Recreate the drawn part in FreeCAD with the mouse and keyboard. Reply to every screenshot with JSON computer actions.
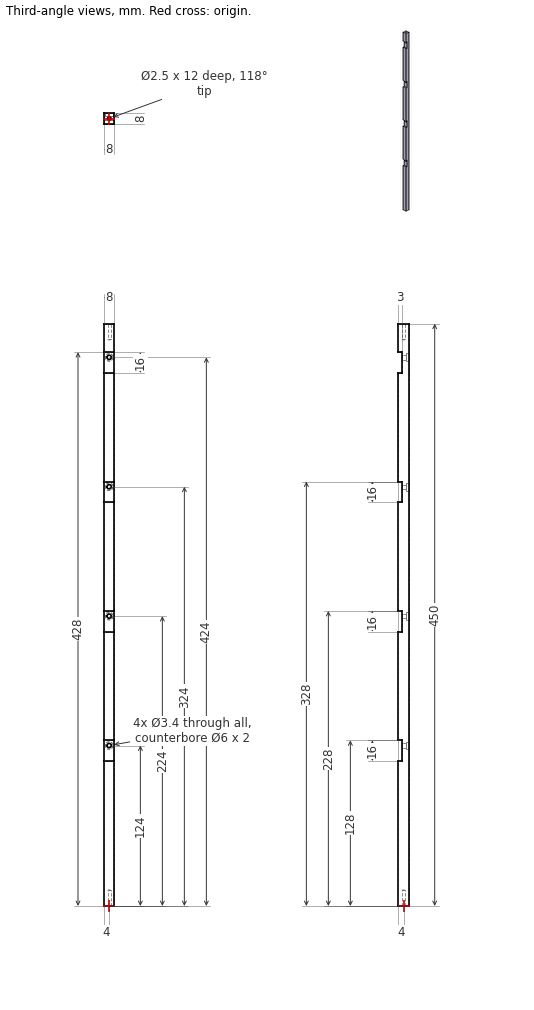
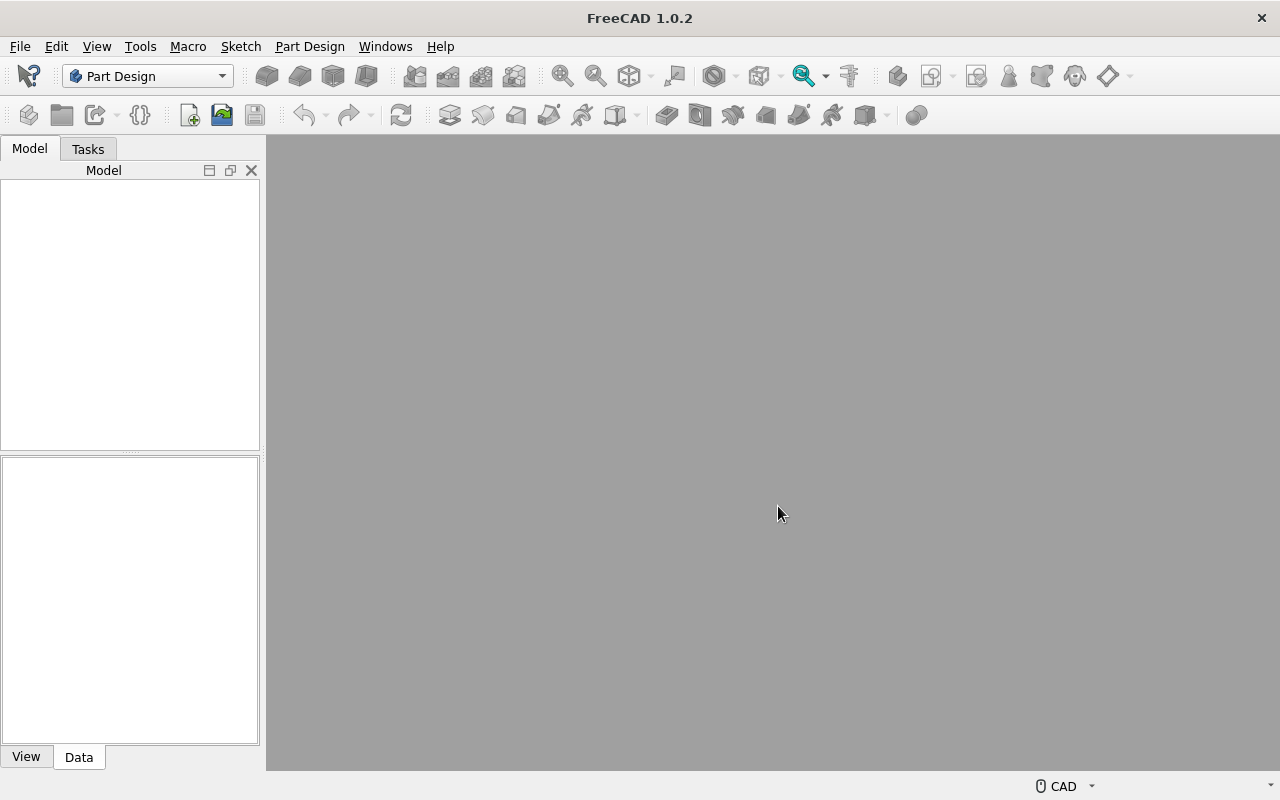
{"action": "key", "text": "ctrl+n"}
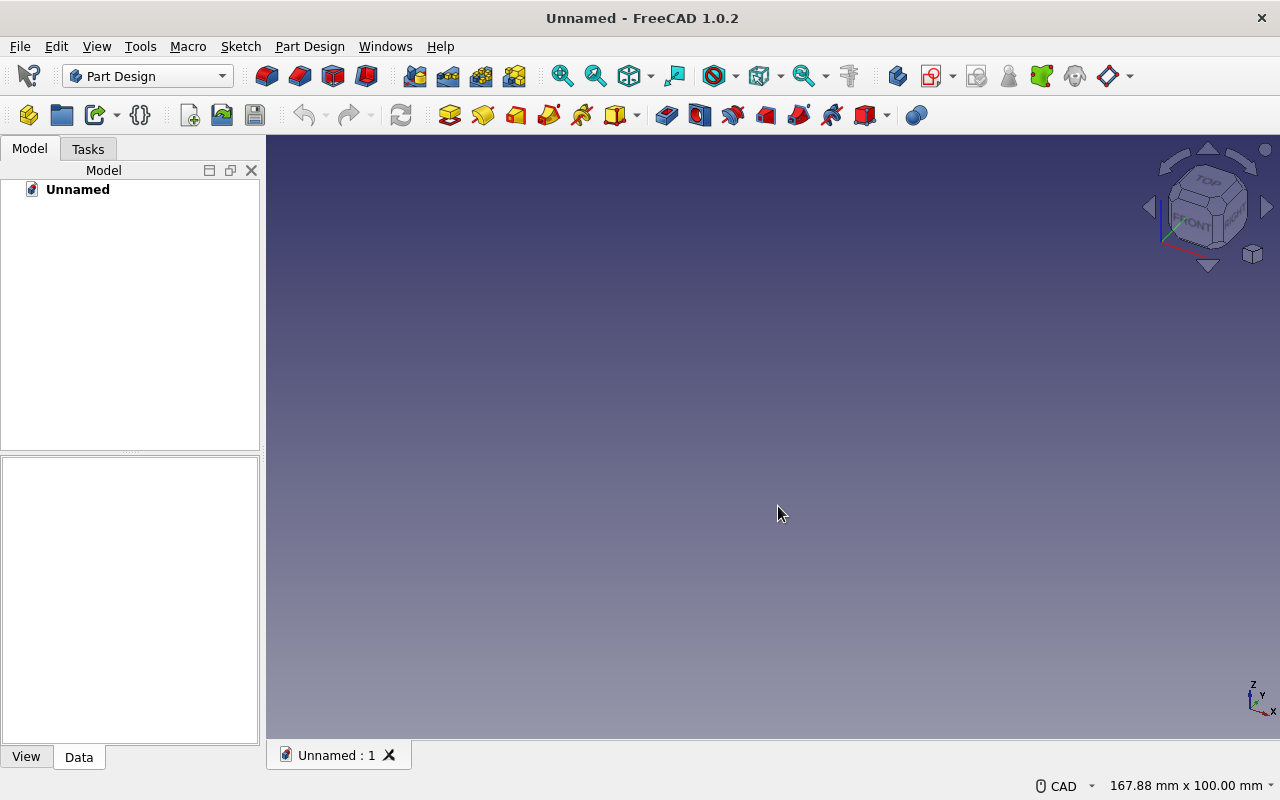
{"action": "left_click", "coordinate": [930, 76]}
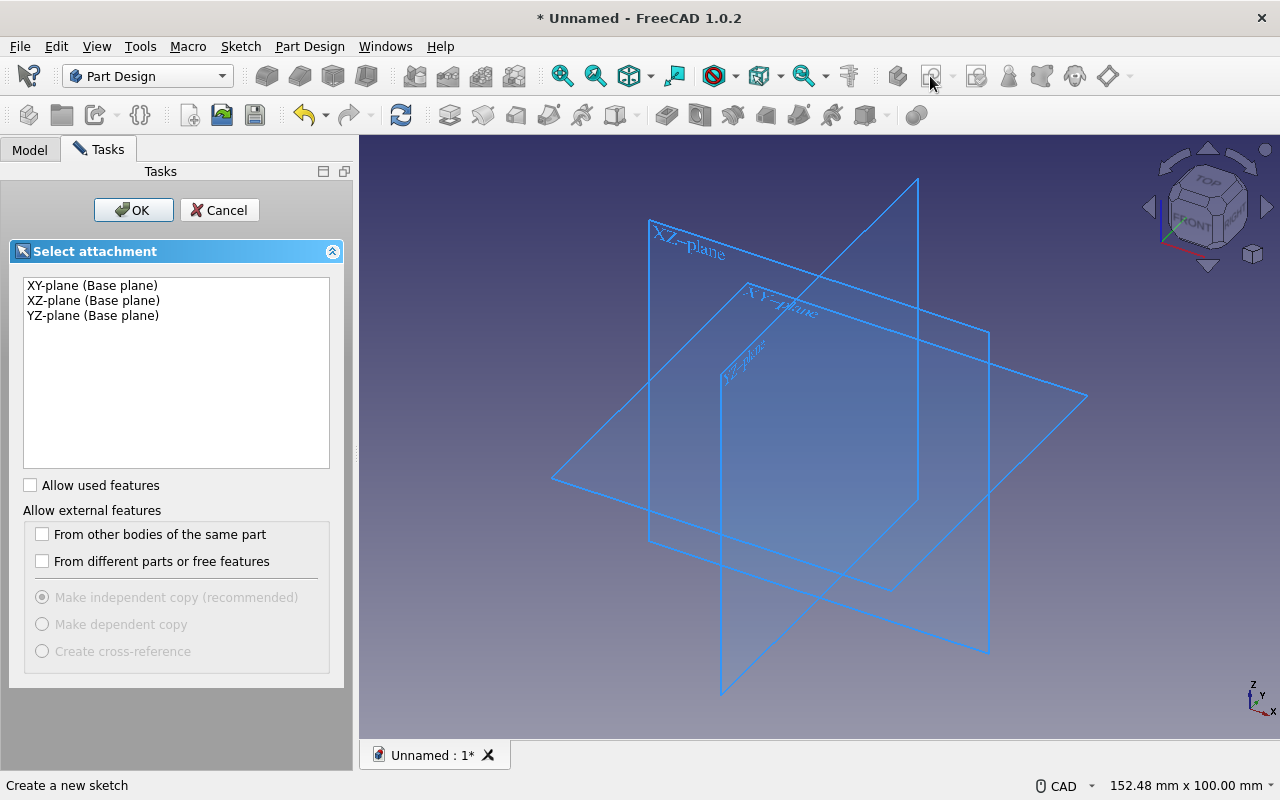
{"action": "left_click", "coordinate": [84, 286]}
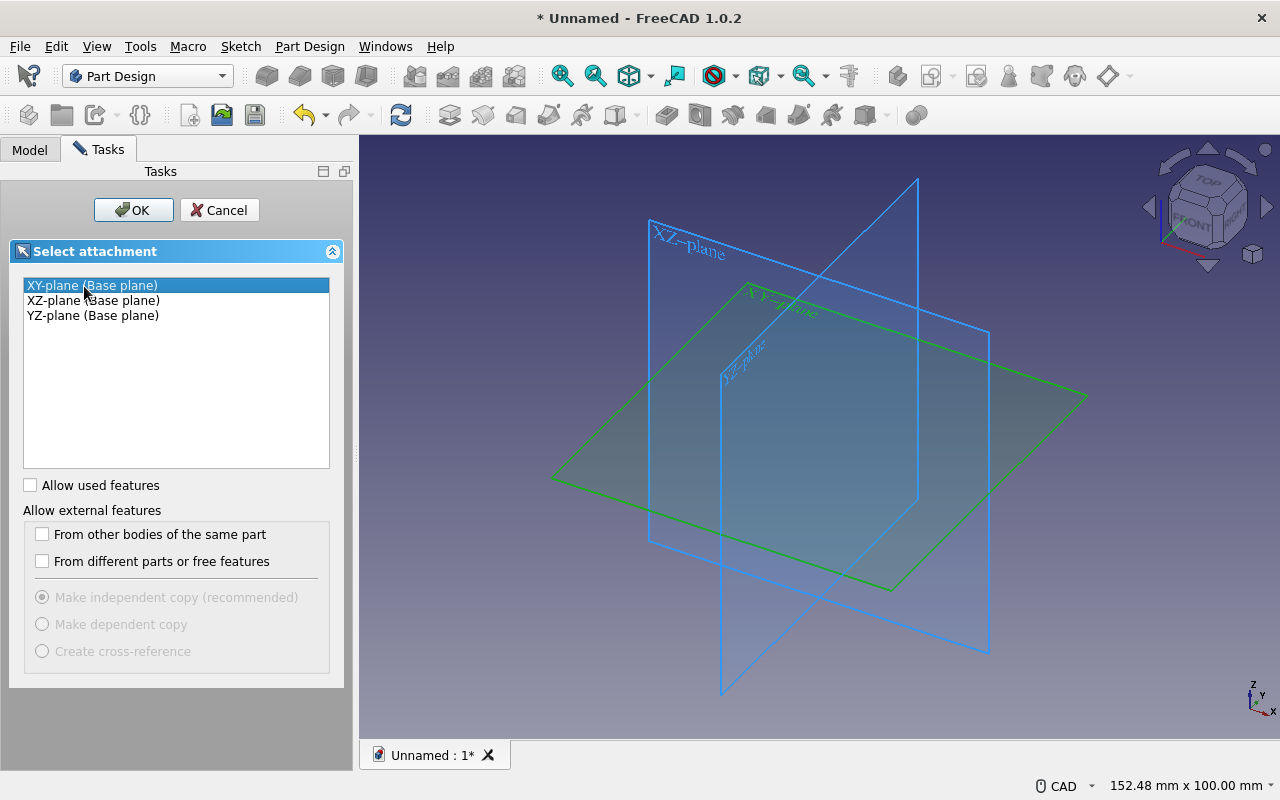
{"action": "left_click", "coordinate": [134, 210]}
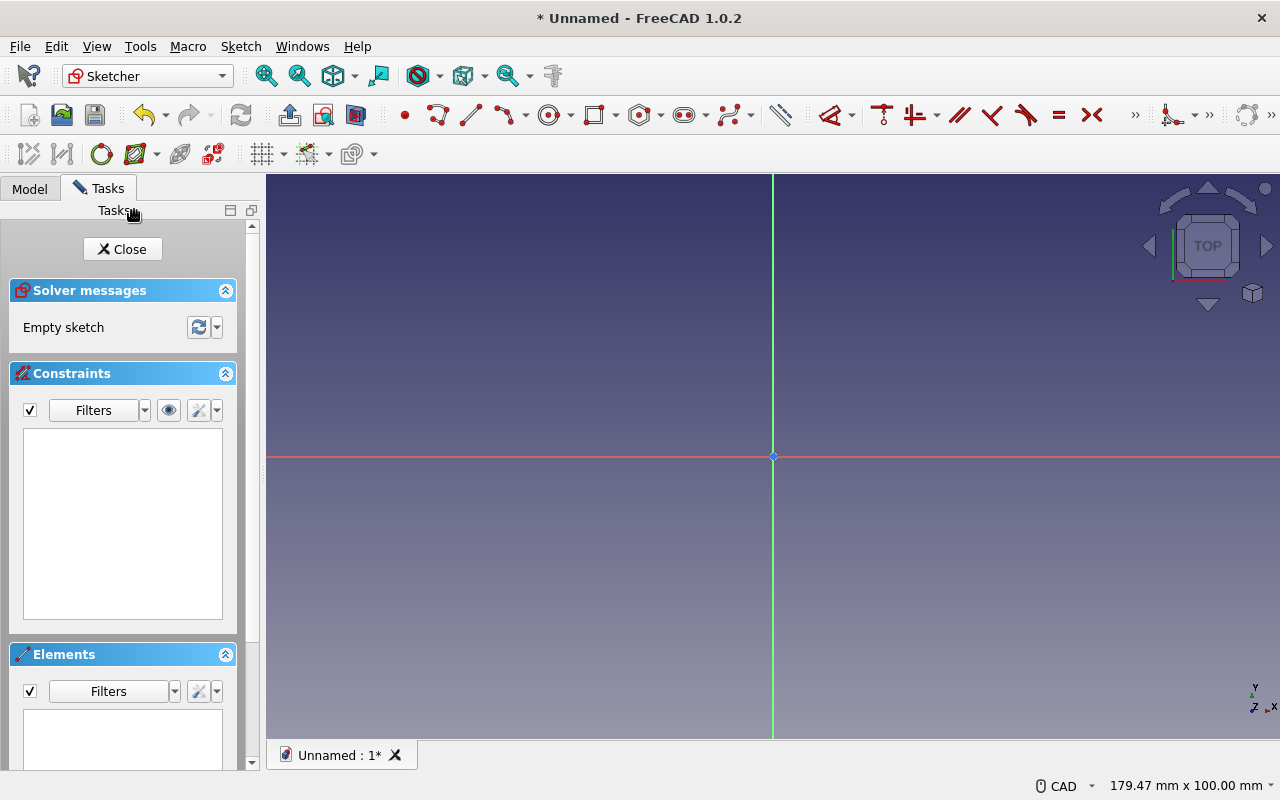
{"action": "scroll", "coordinate": [784, 456], "scroll_direction": "up", "scroll_amount": 10}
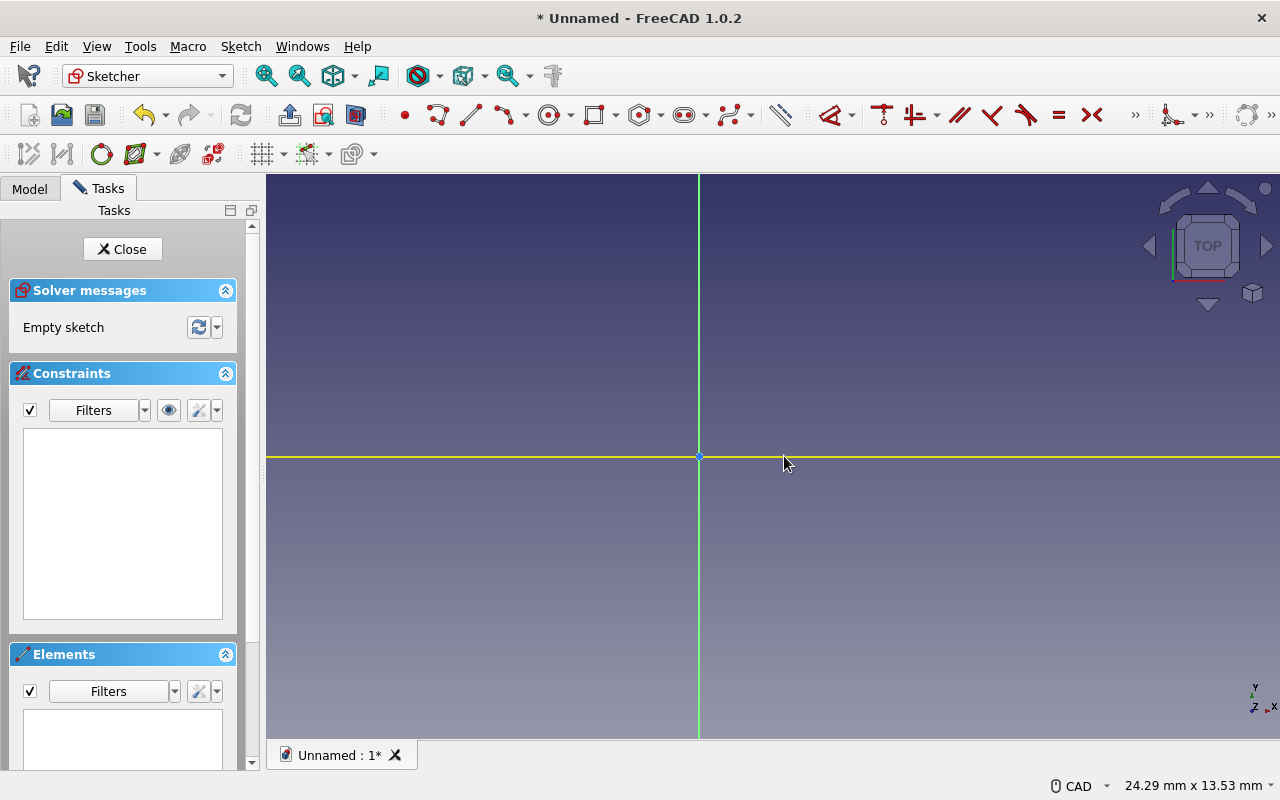
{"action": "key", "text": "g v"}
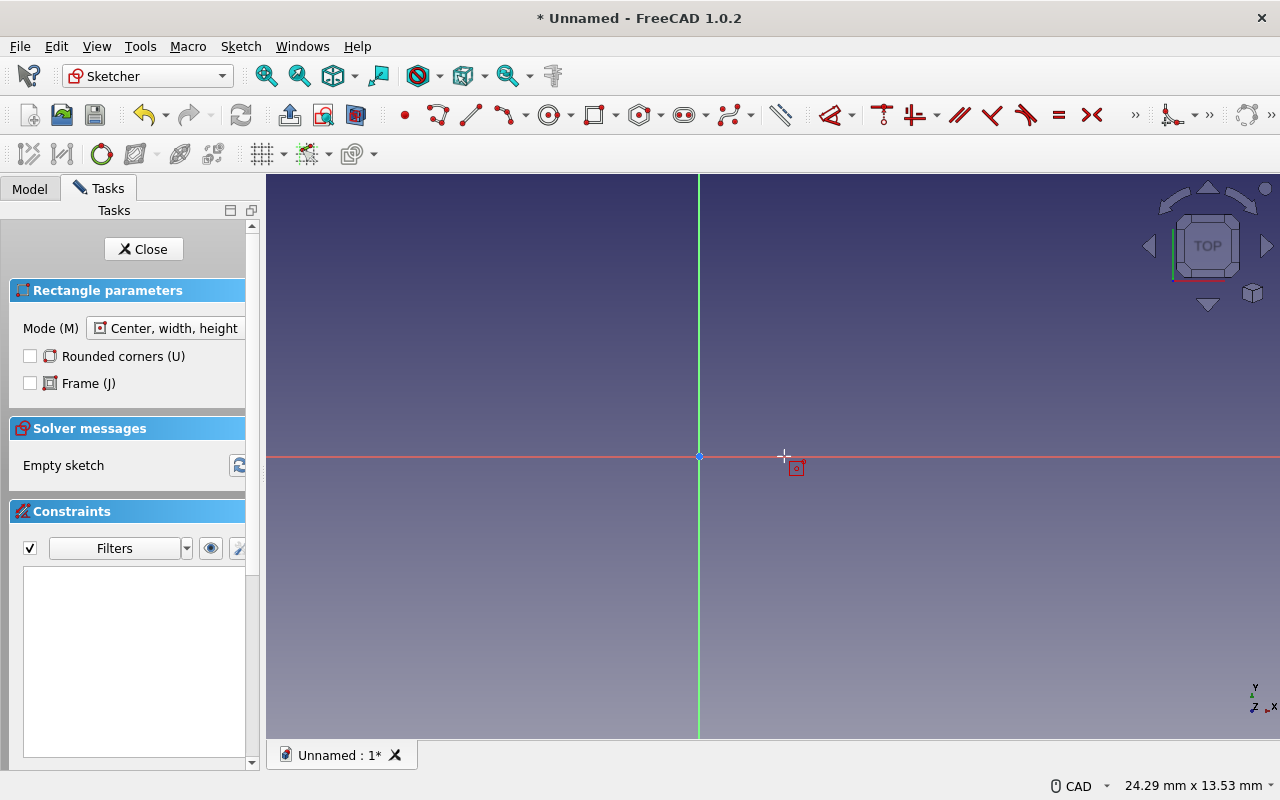
{"action": "left_click", "coordinate": [699, 456]}
{"action": "mouse_move", "coordinate": [866, 290]}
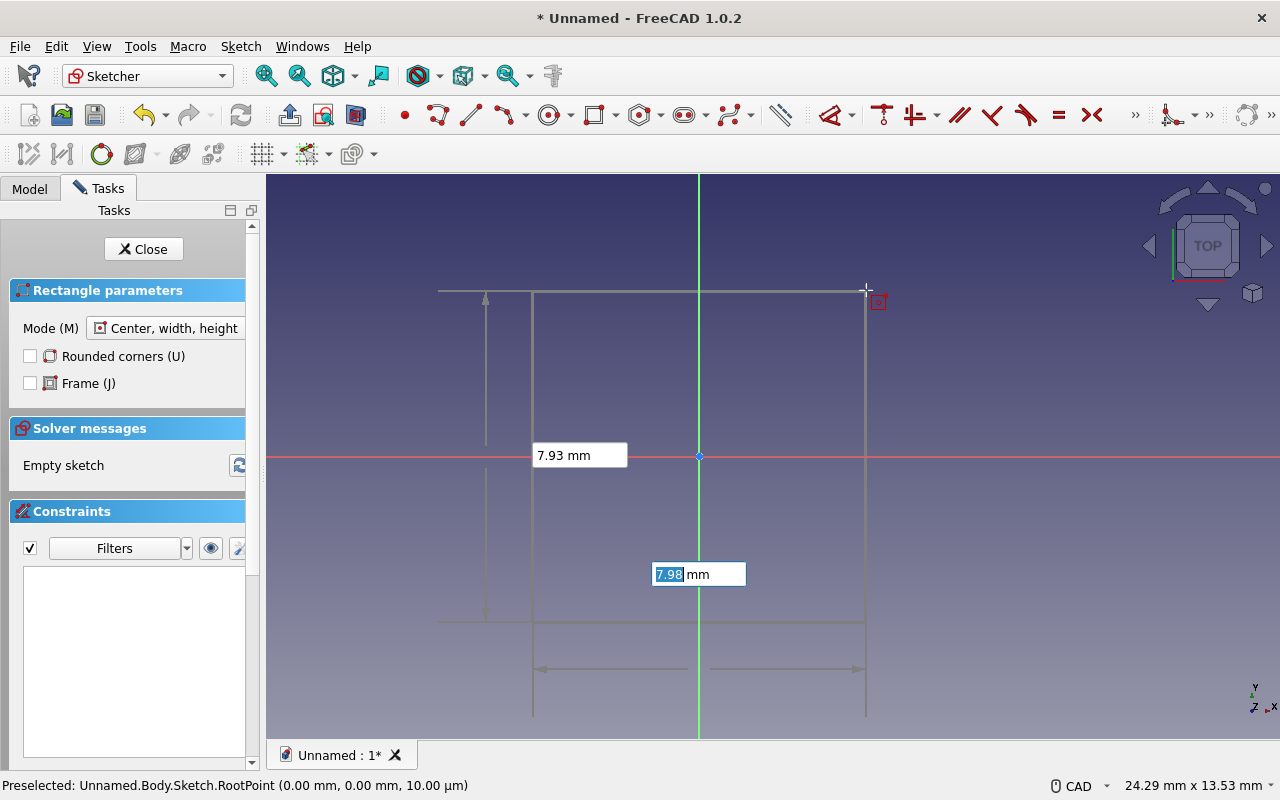
{"action": "type", "text": "8"}
{"action": "key", "text": "Tab"}
{"action": "type", "text": "8"}
{"action": "key", "text": "Return"}
{"action": "key", "text": "Escape"}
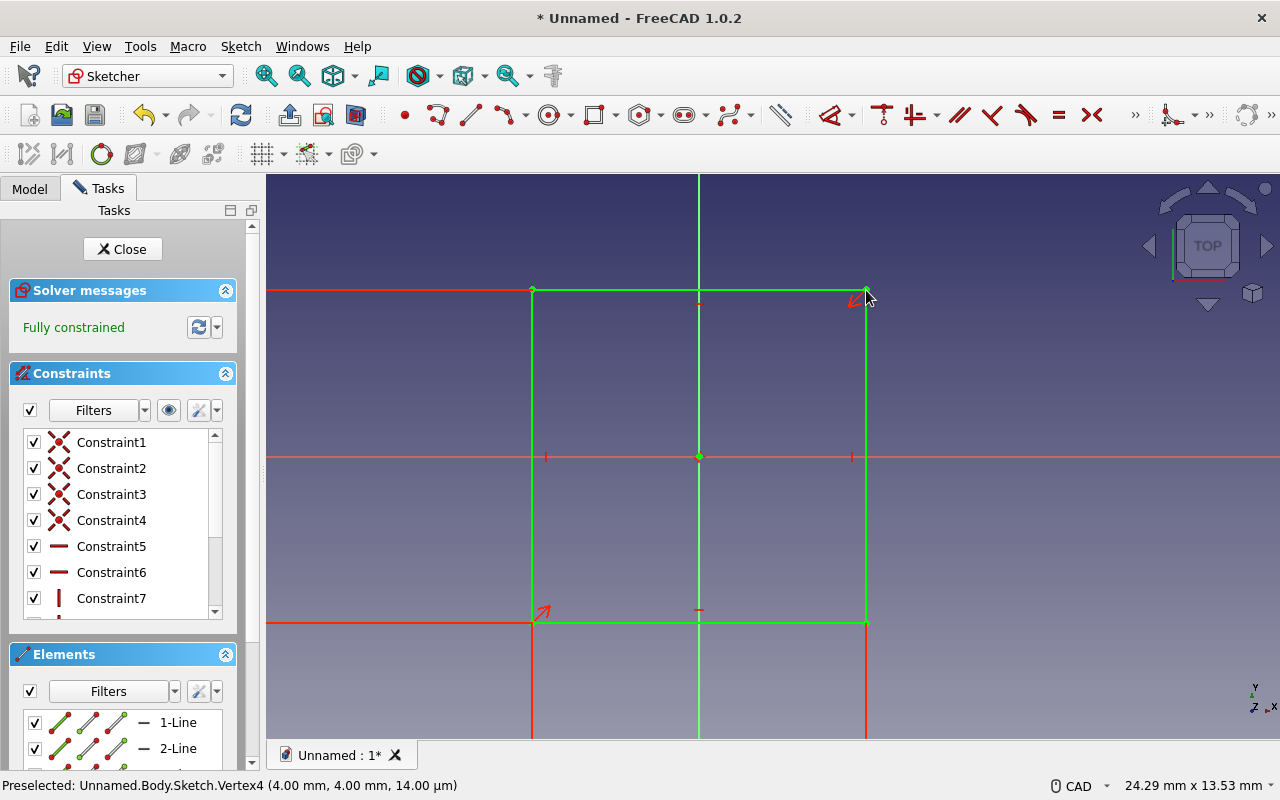
{"action": "left_click", "coordinate": [123, 249]}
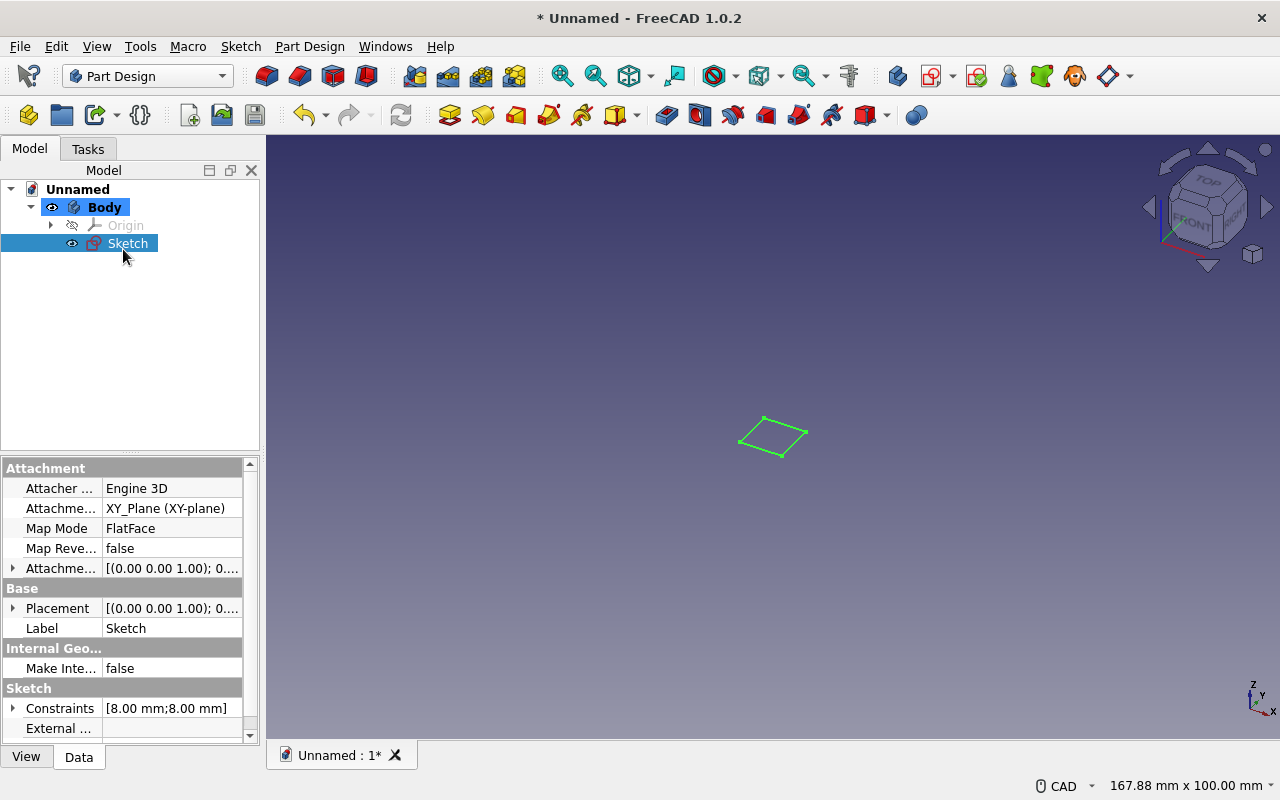
{"action": "left_click", "coordinate": [450, 116]}